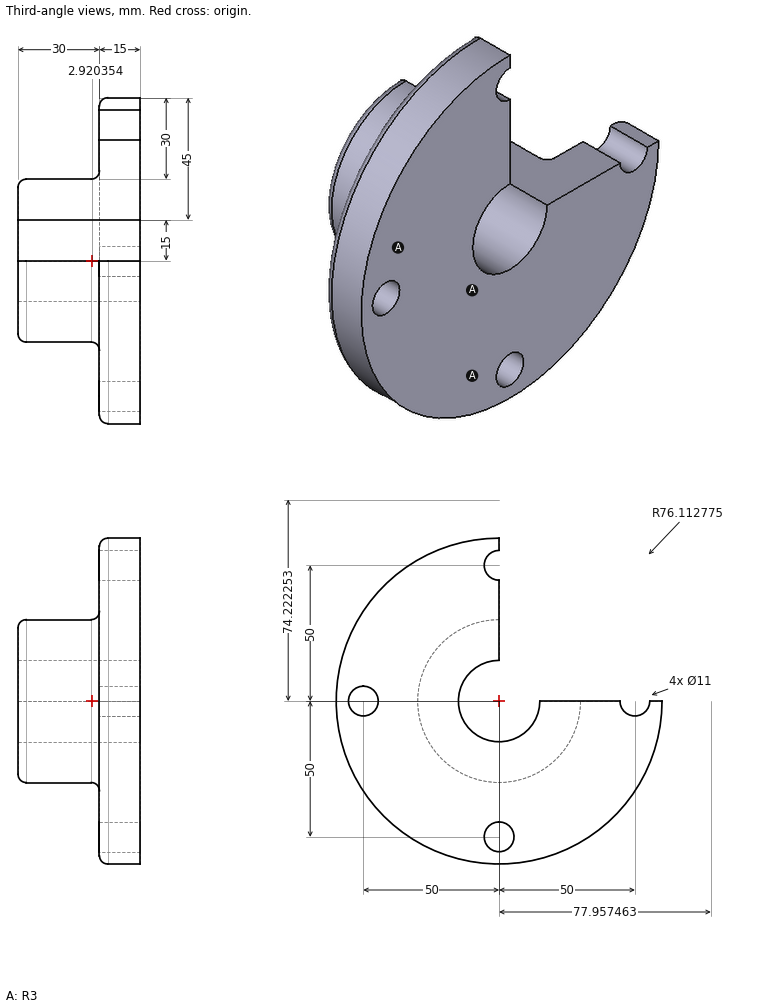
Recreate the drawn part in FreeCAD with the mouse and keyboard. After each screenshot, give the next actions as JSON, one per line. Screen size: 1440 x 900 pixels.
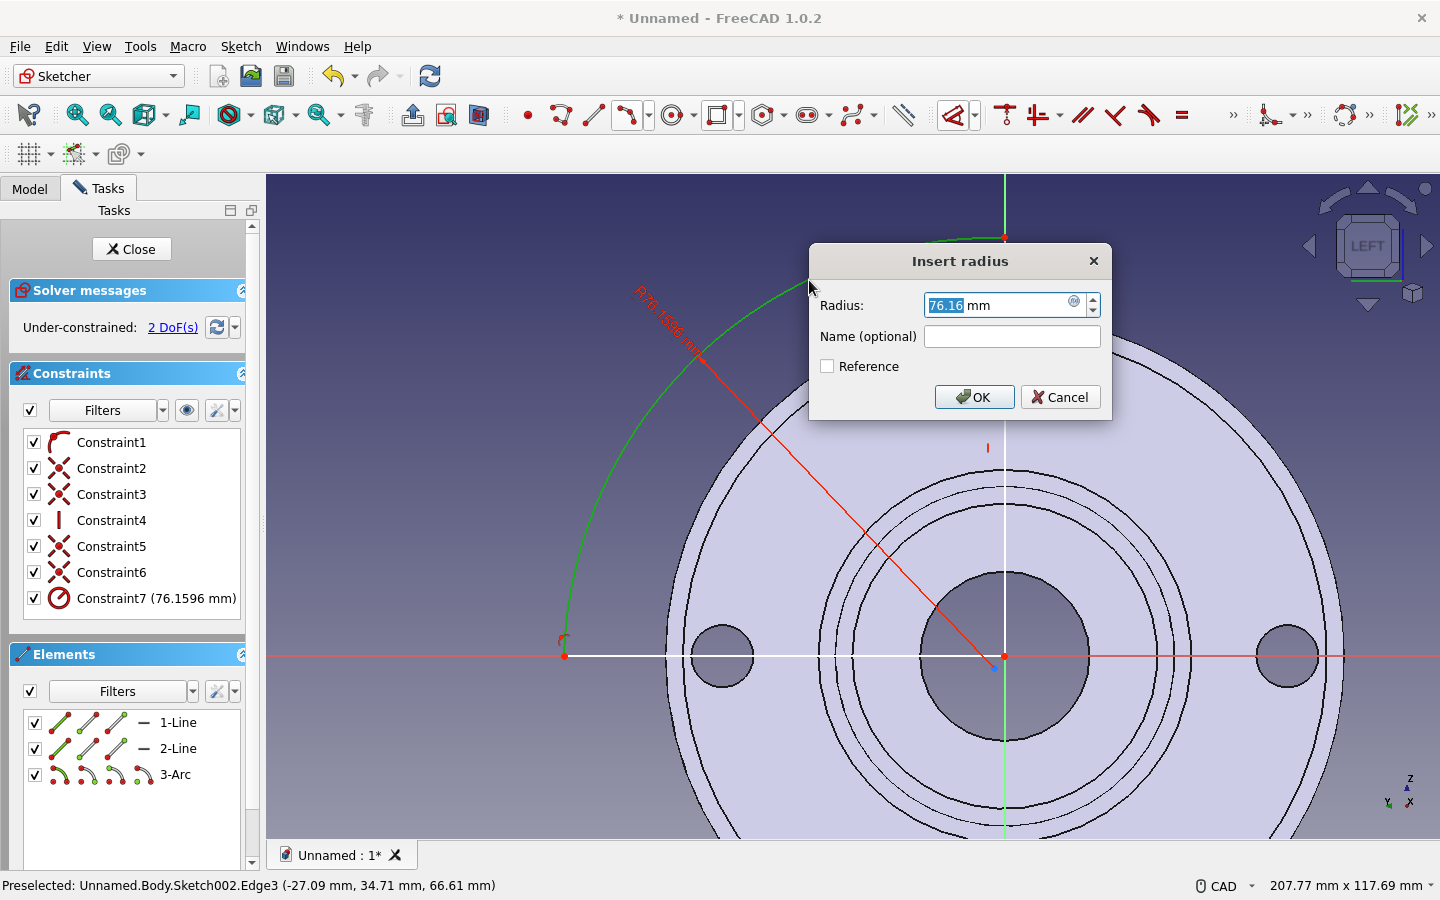
{"action": "type", "text": "76.112775"}
{"action": "key", "text": "Return"}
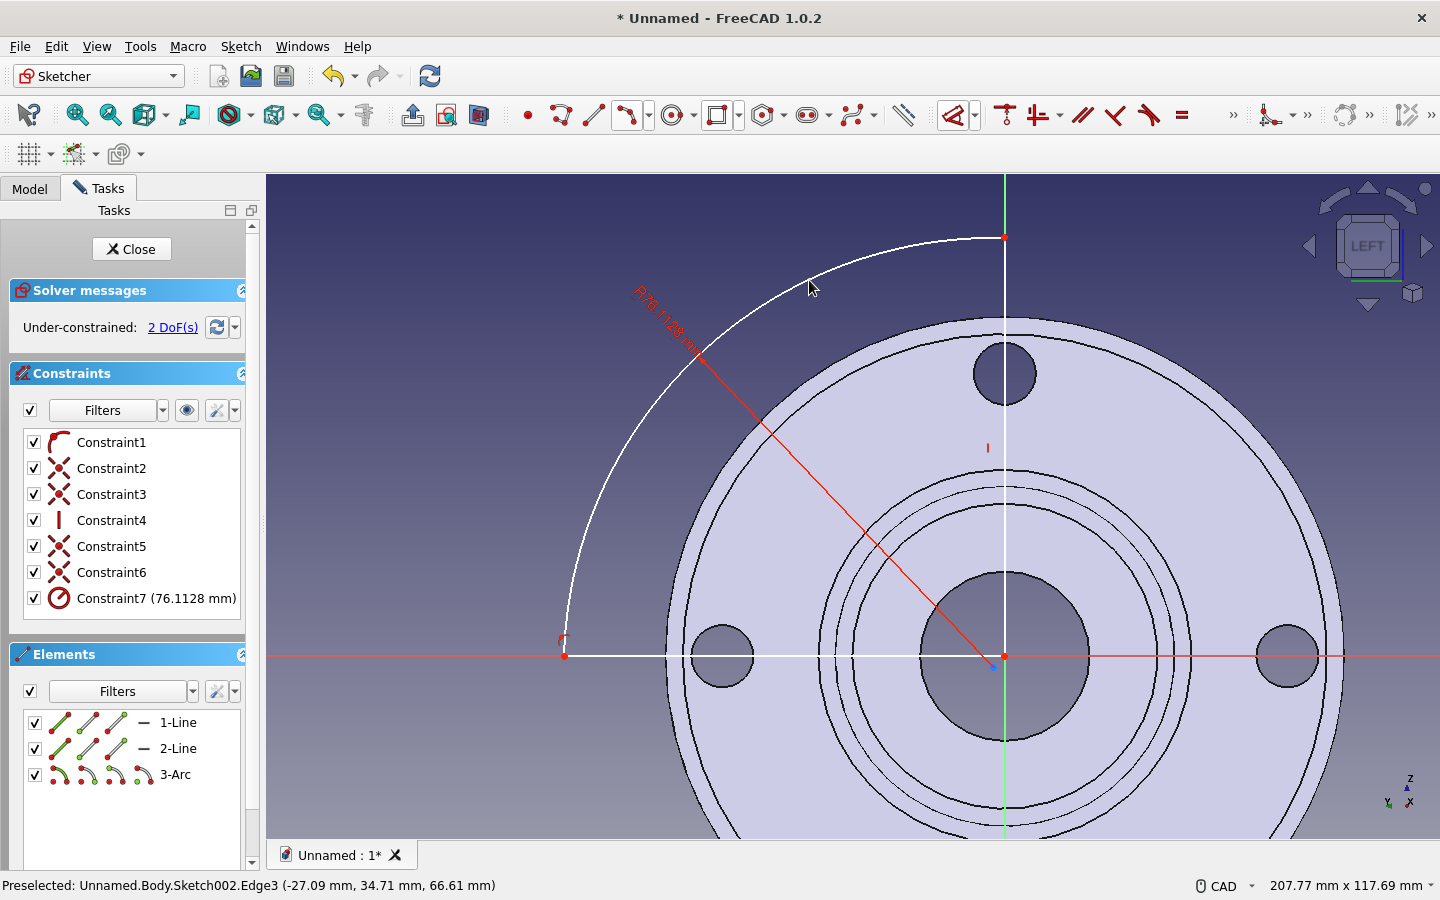
{"action": "left_click", "coordinate": [696, 656]}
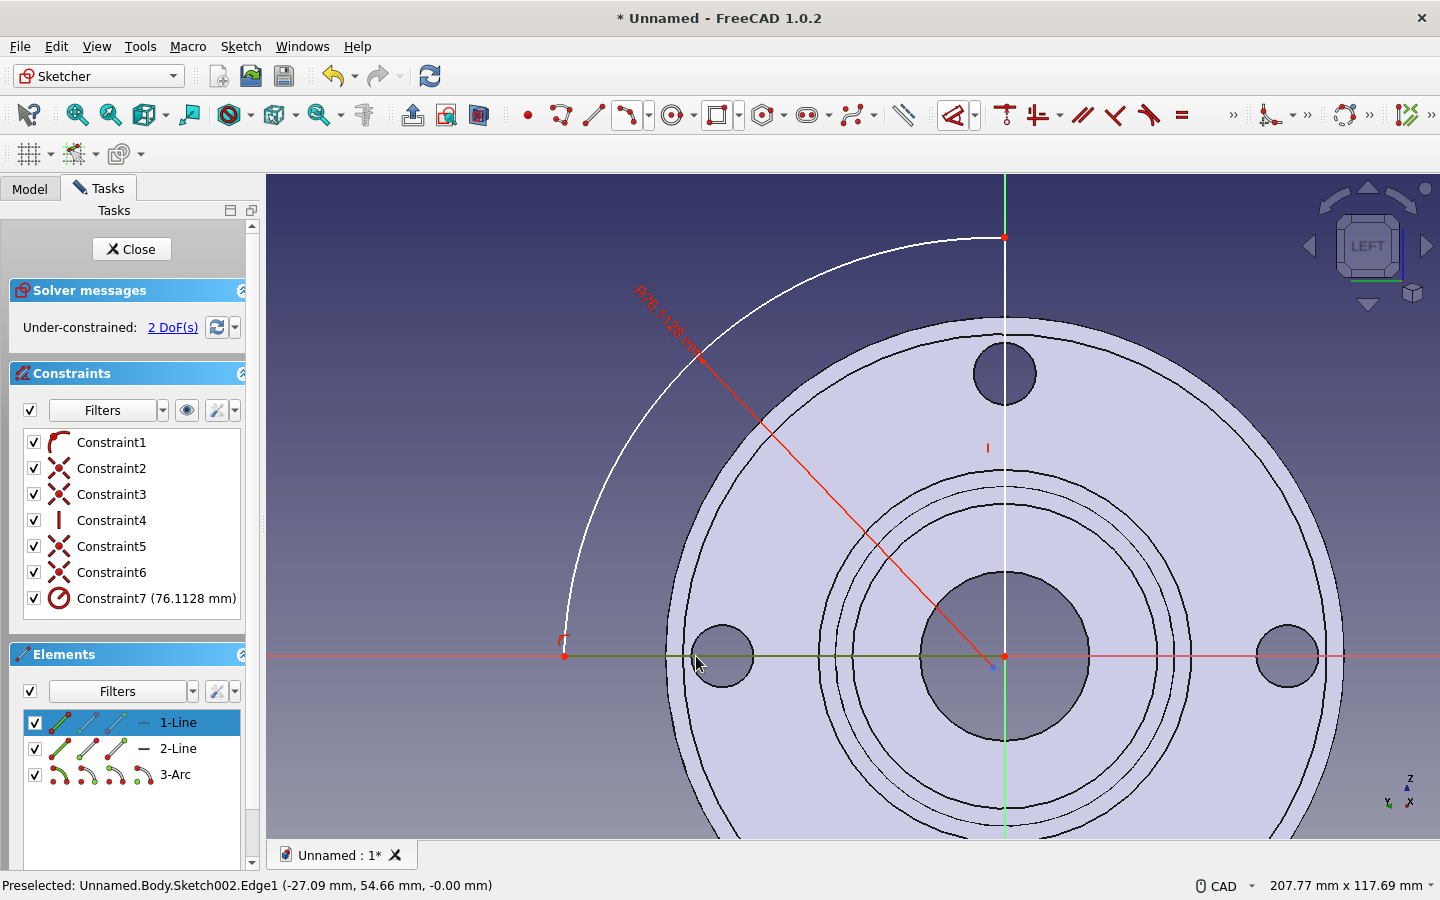
{"action": "key", "text": "l"}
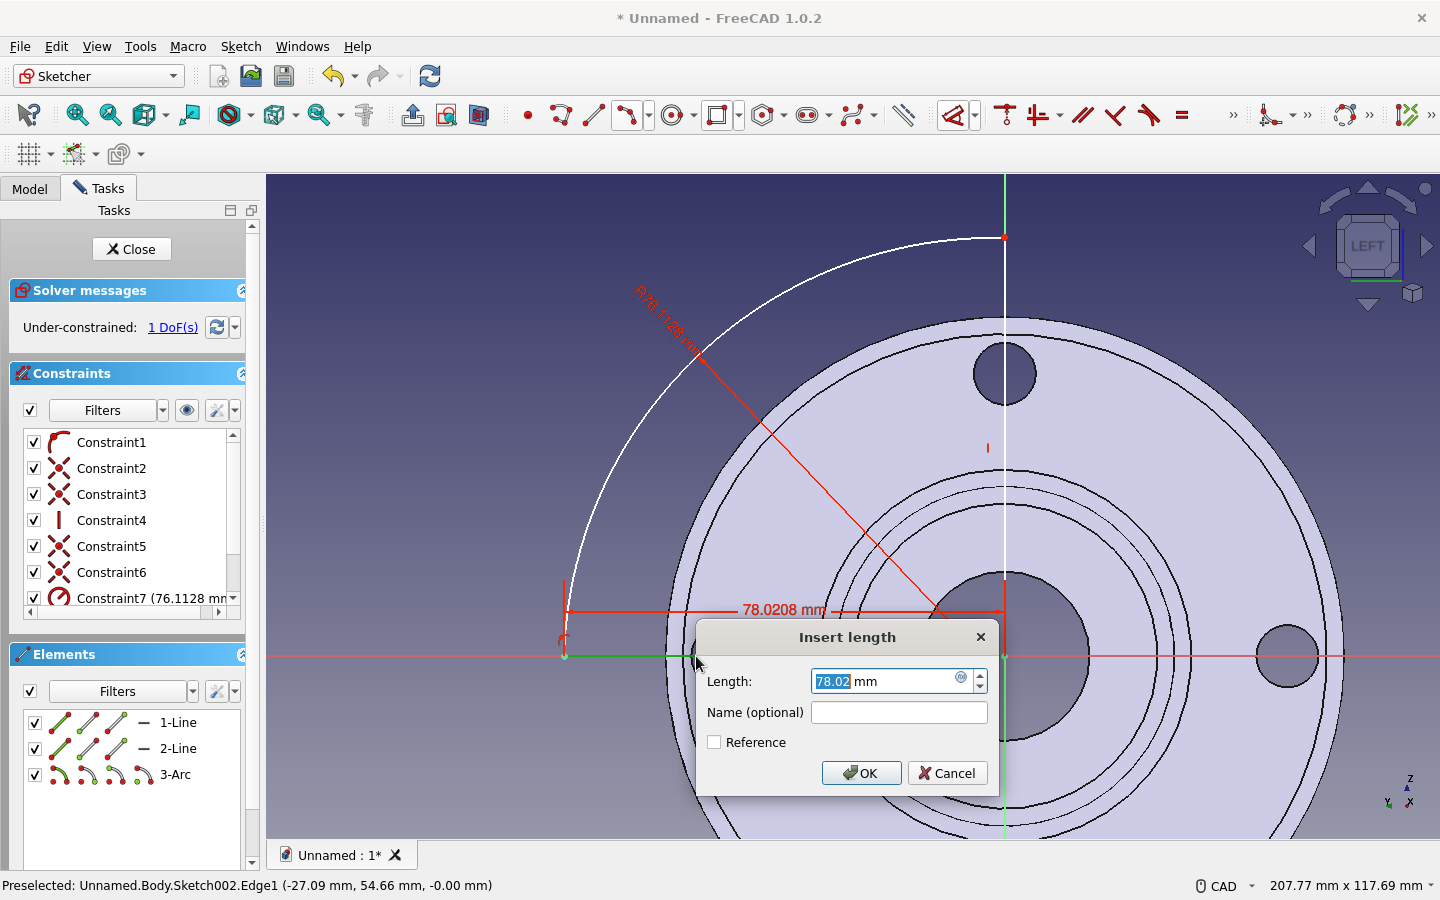
{"action": "type", "text": "77.957463"}
{"action": "key", "text": "Return"}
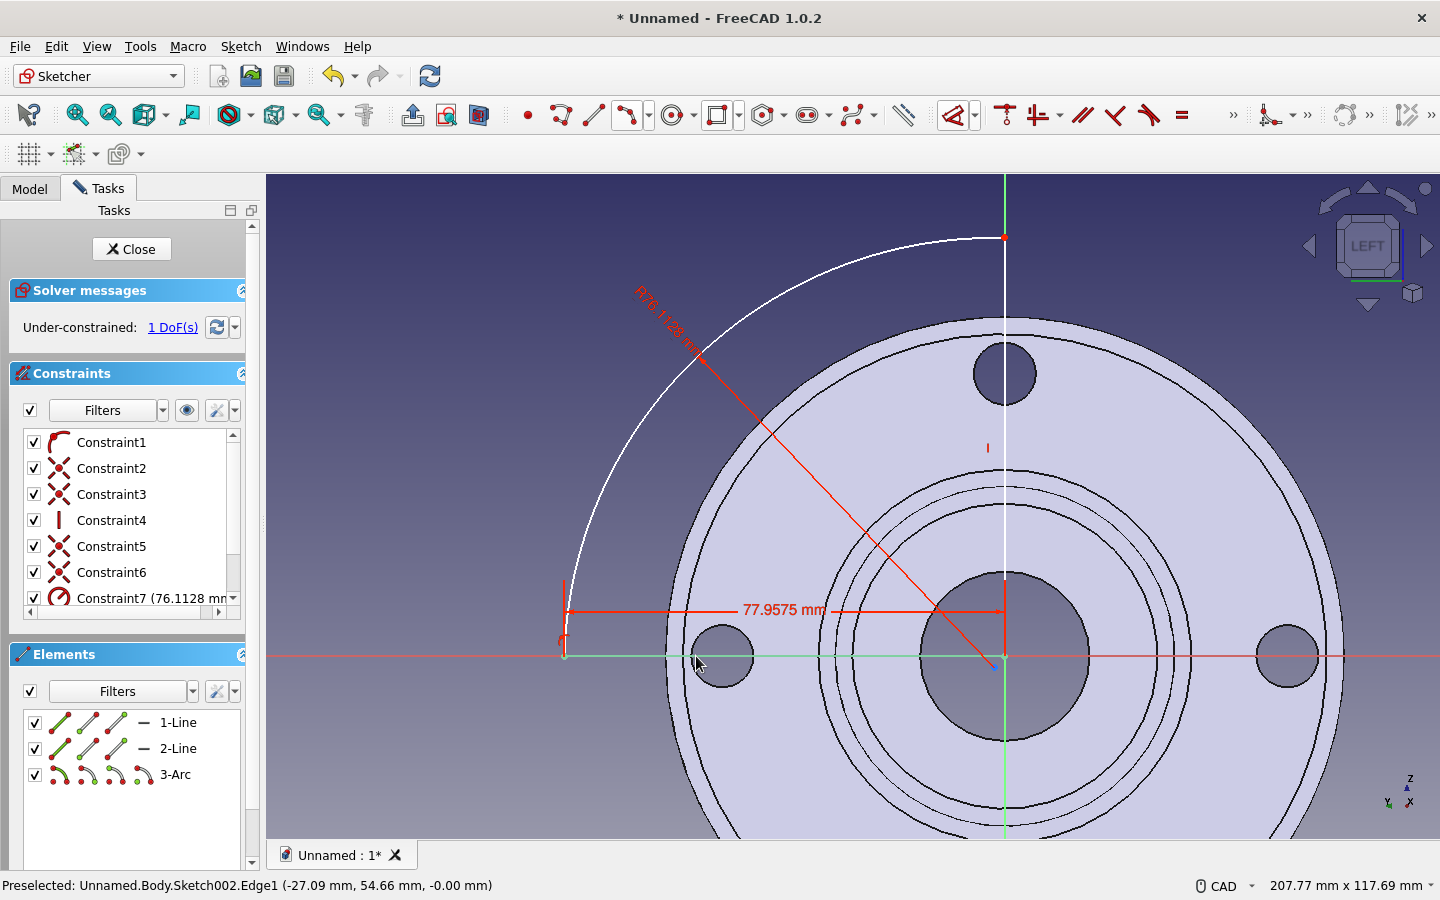
{"action": "left_click", "coordinate": [1005, 531]}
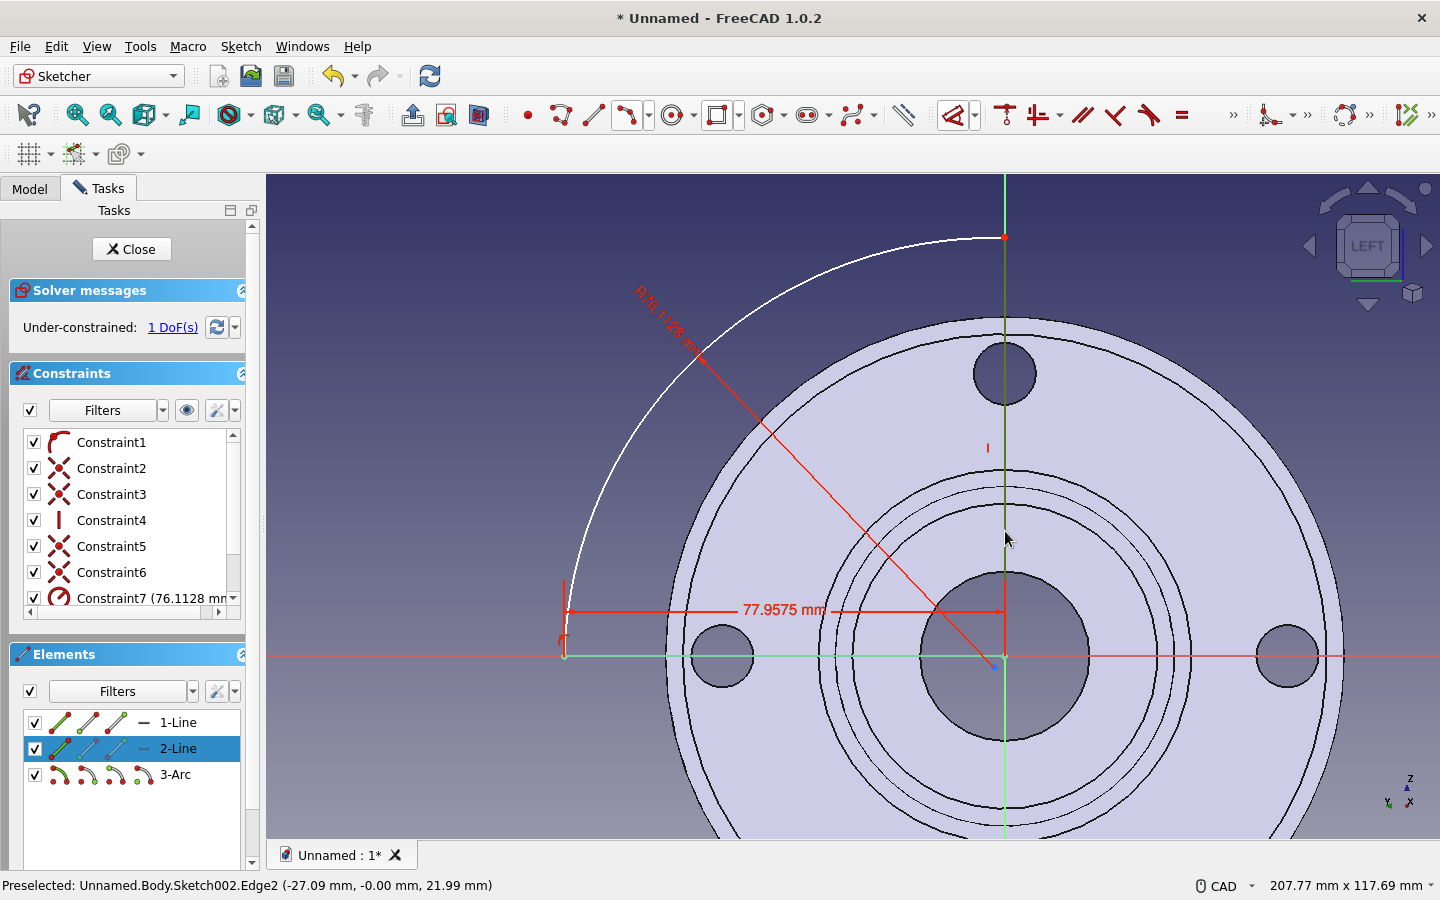
{"action": "left_click", "coordinate": [974, 116]}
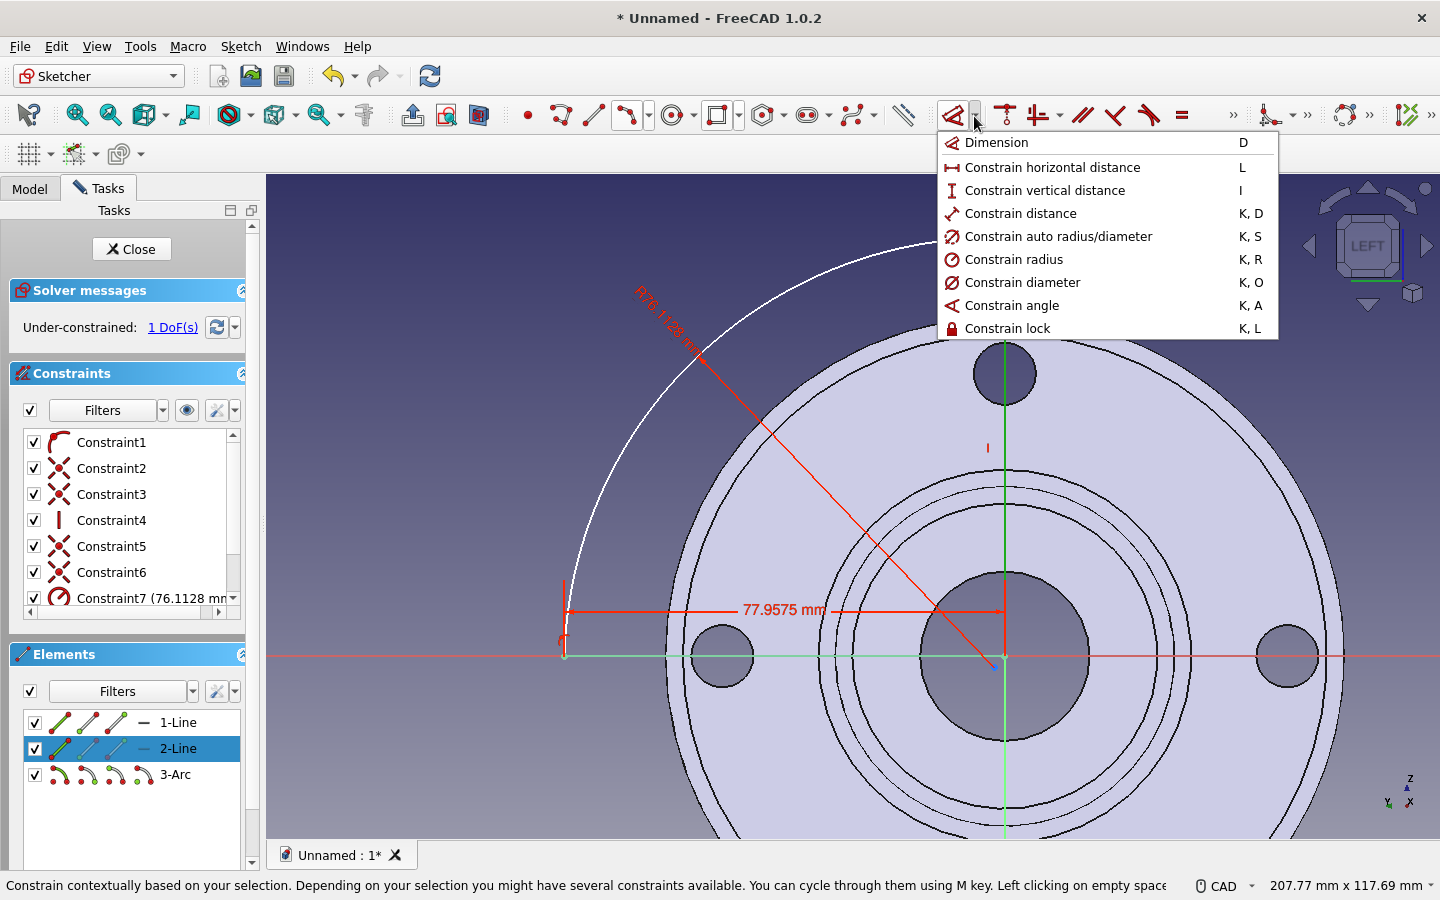
{"action": "left_click", "coordinate": [1108, 190]}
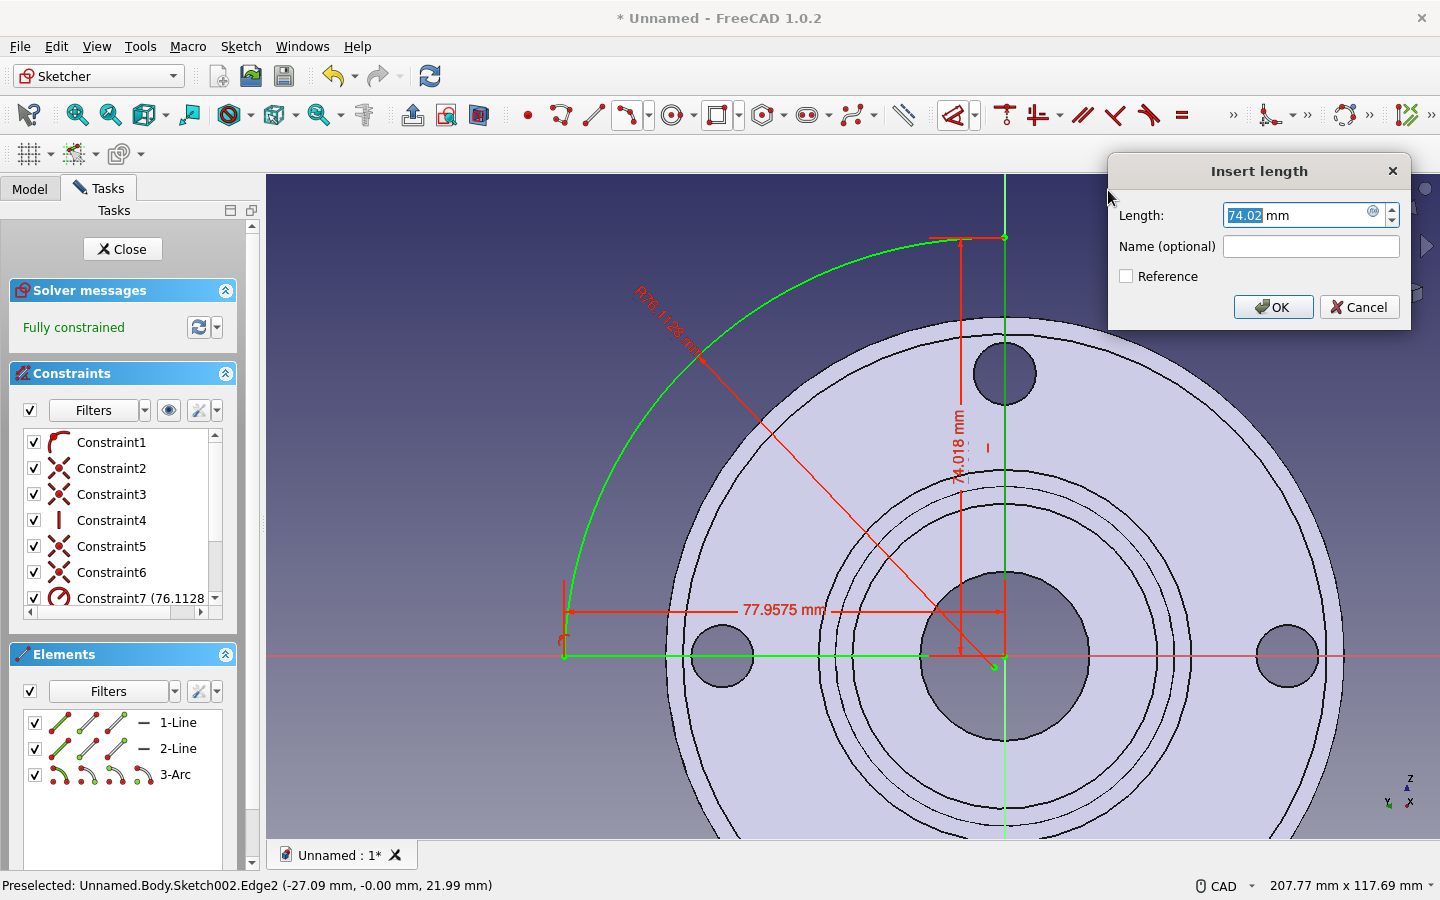
{"action": "type", "text": "74.222253"}
{"action": "key", "text": "Return"}